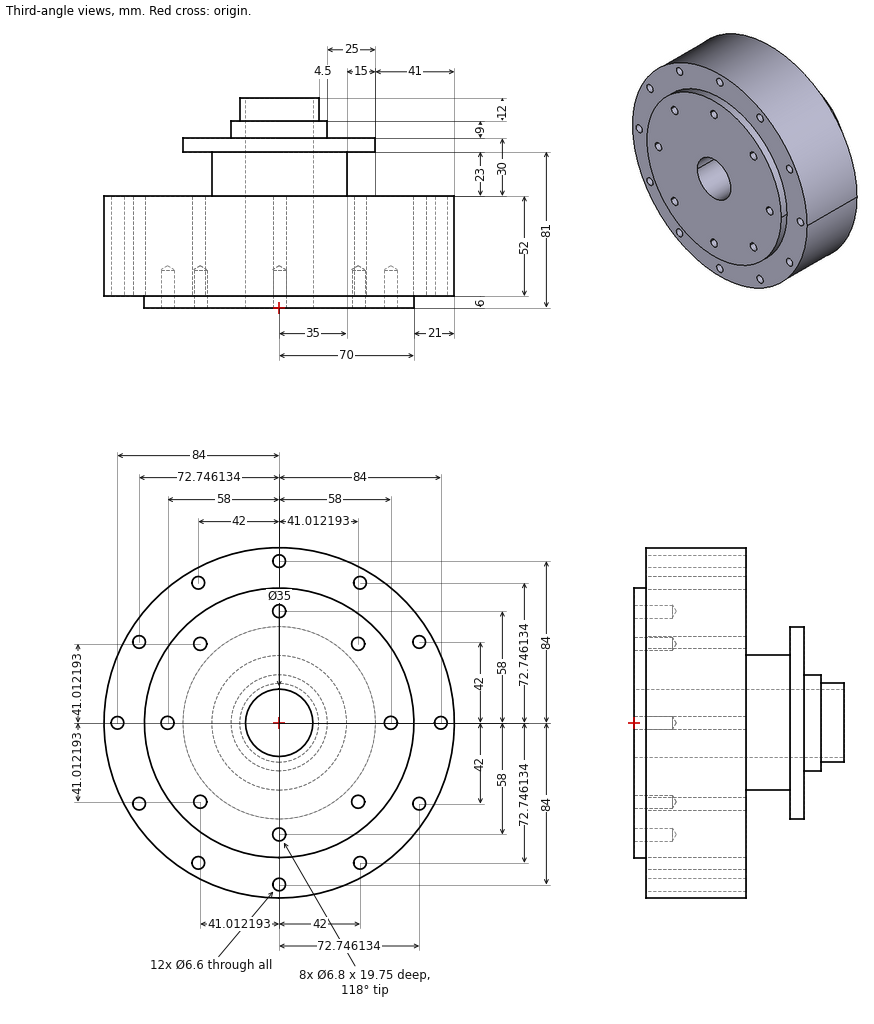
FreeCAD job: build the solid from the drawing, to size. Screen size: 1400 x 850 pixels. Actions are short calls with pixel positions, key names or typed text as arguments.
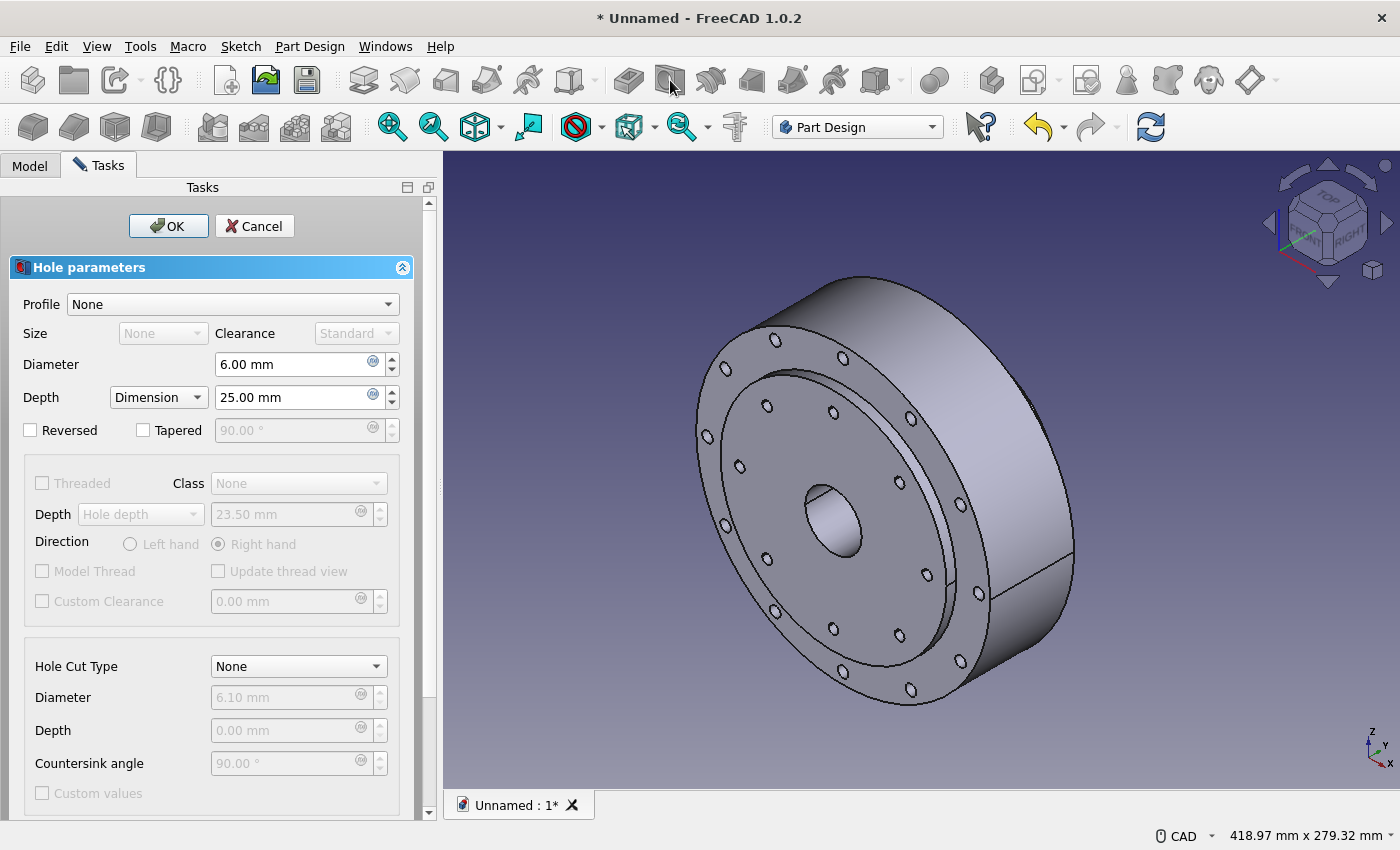
triple_click(300, 364)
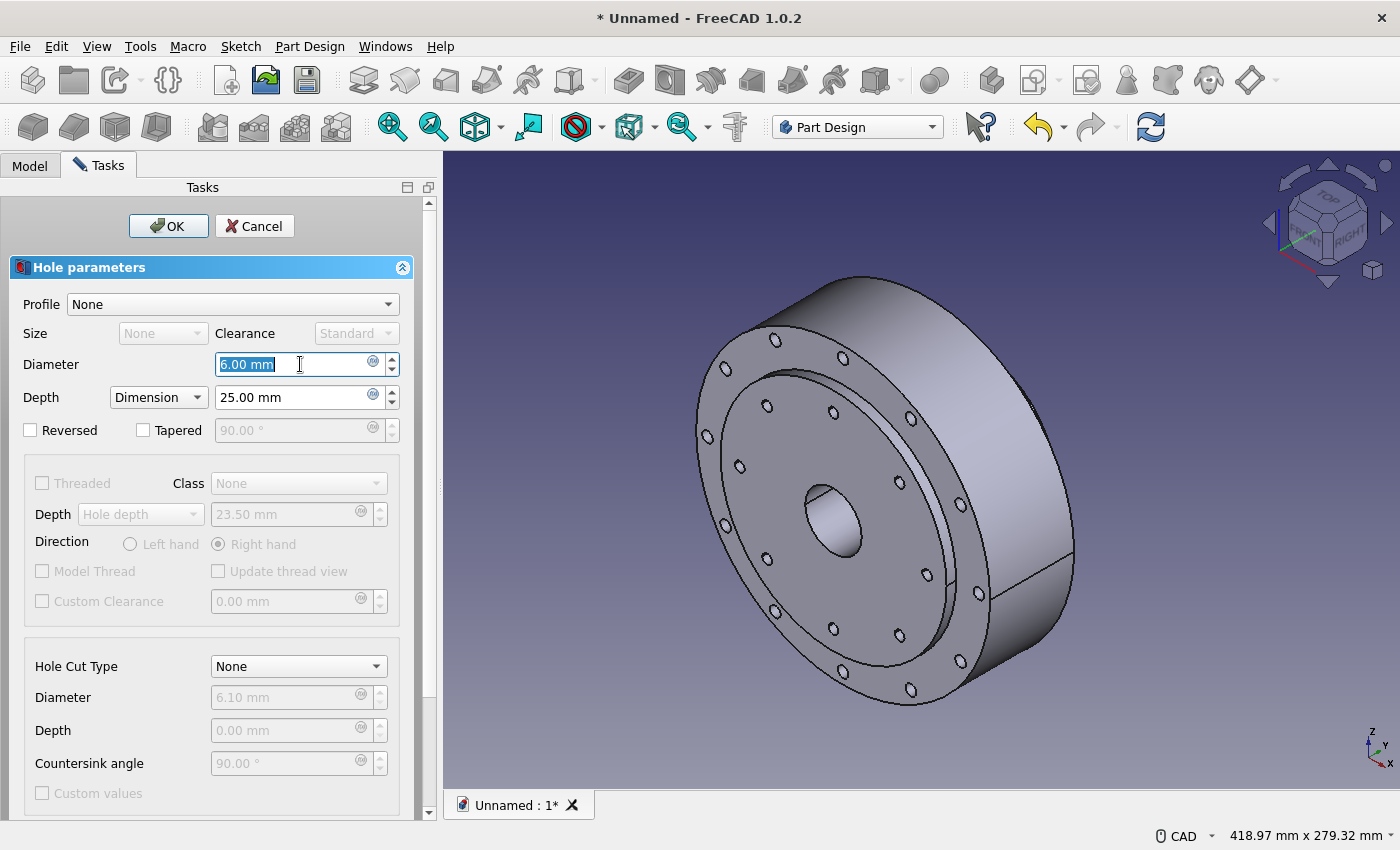
text(6.8)
key(Tab)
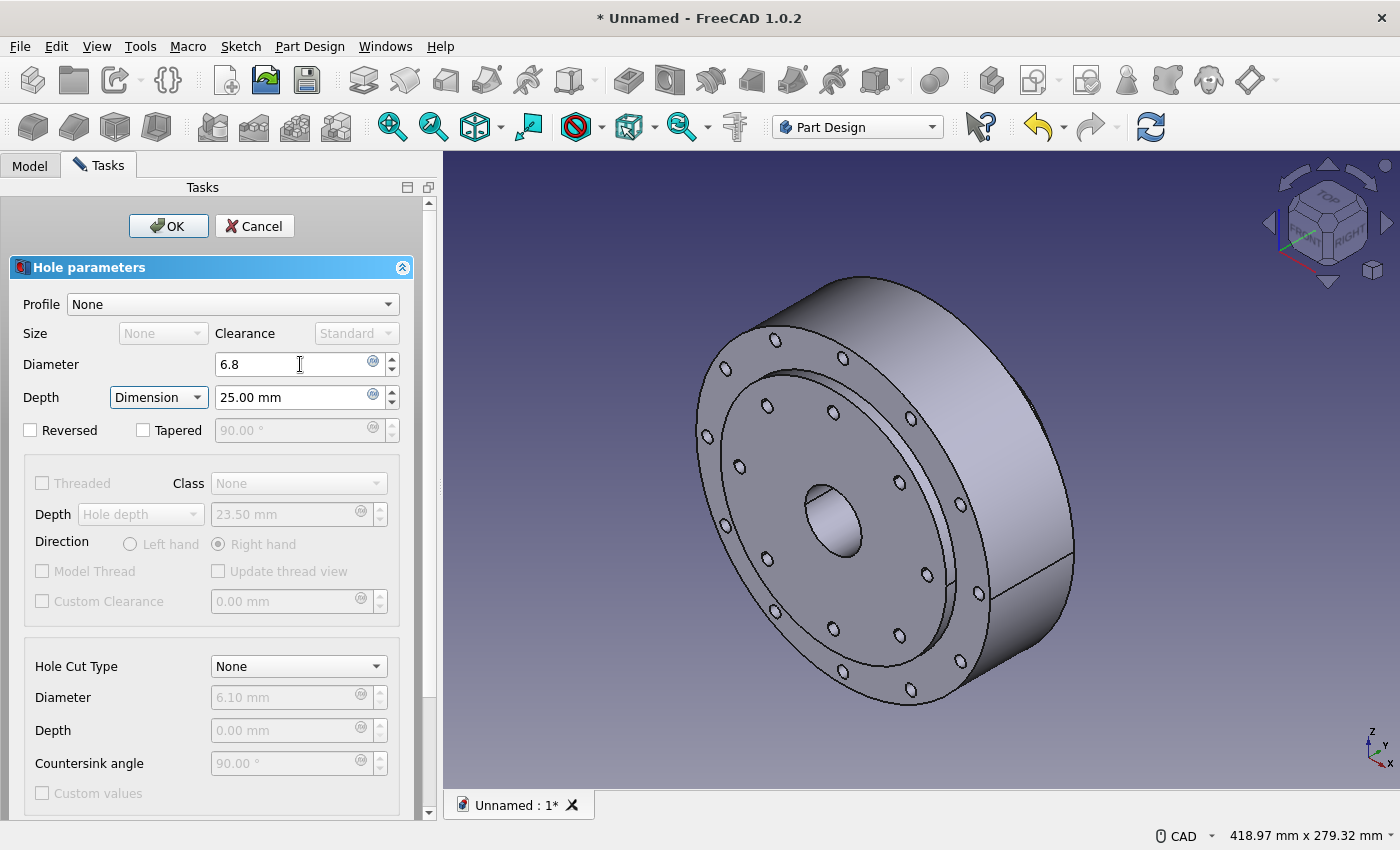
triple_click(300, 398)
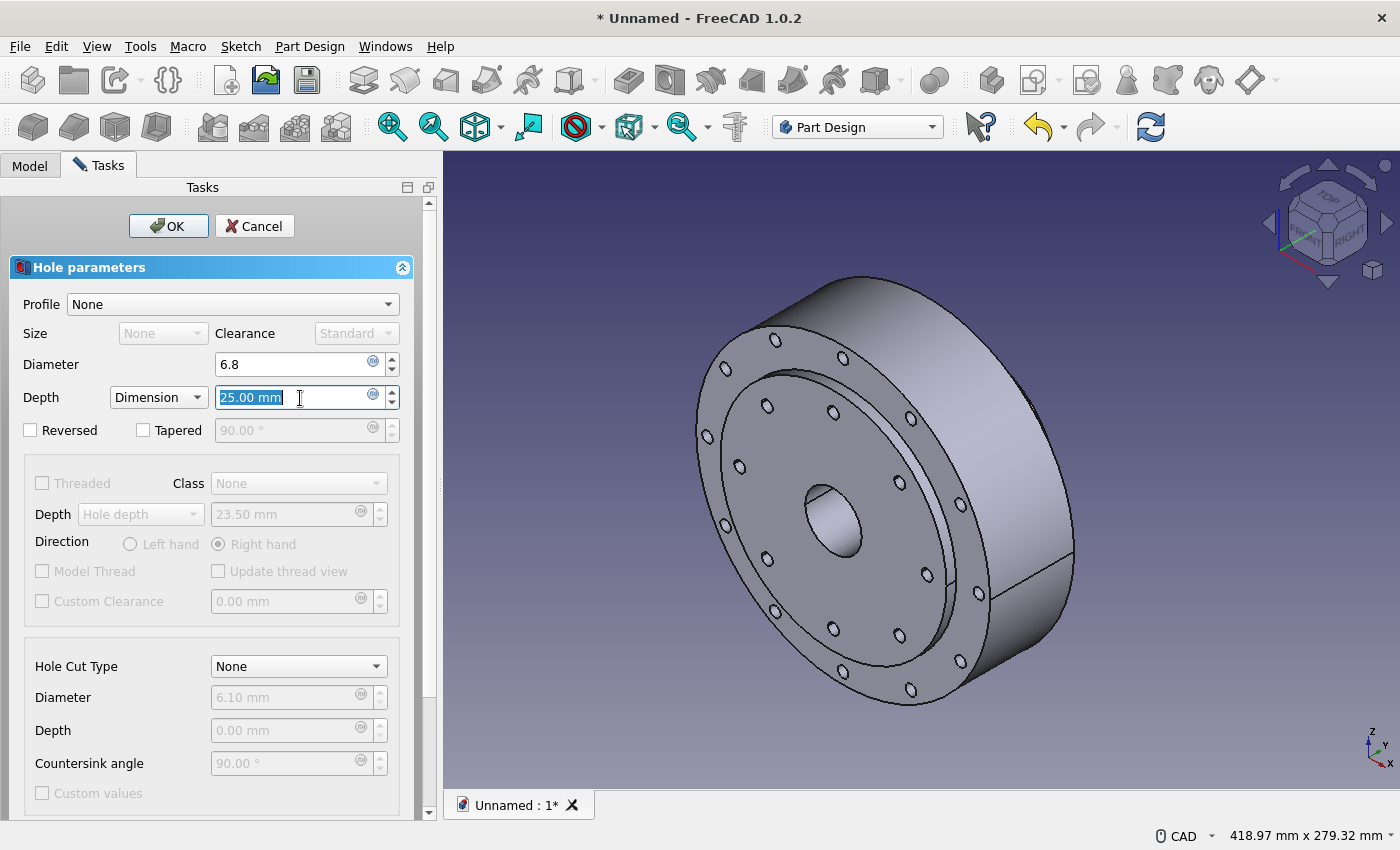
text(19.75)
key(Tab)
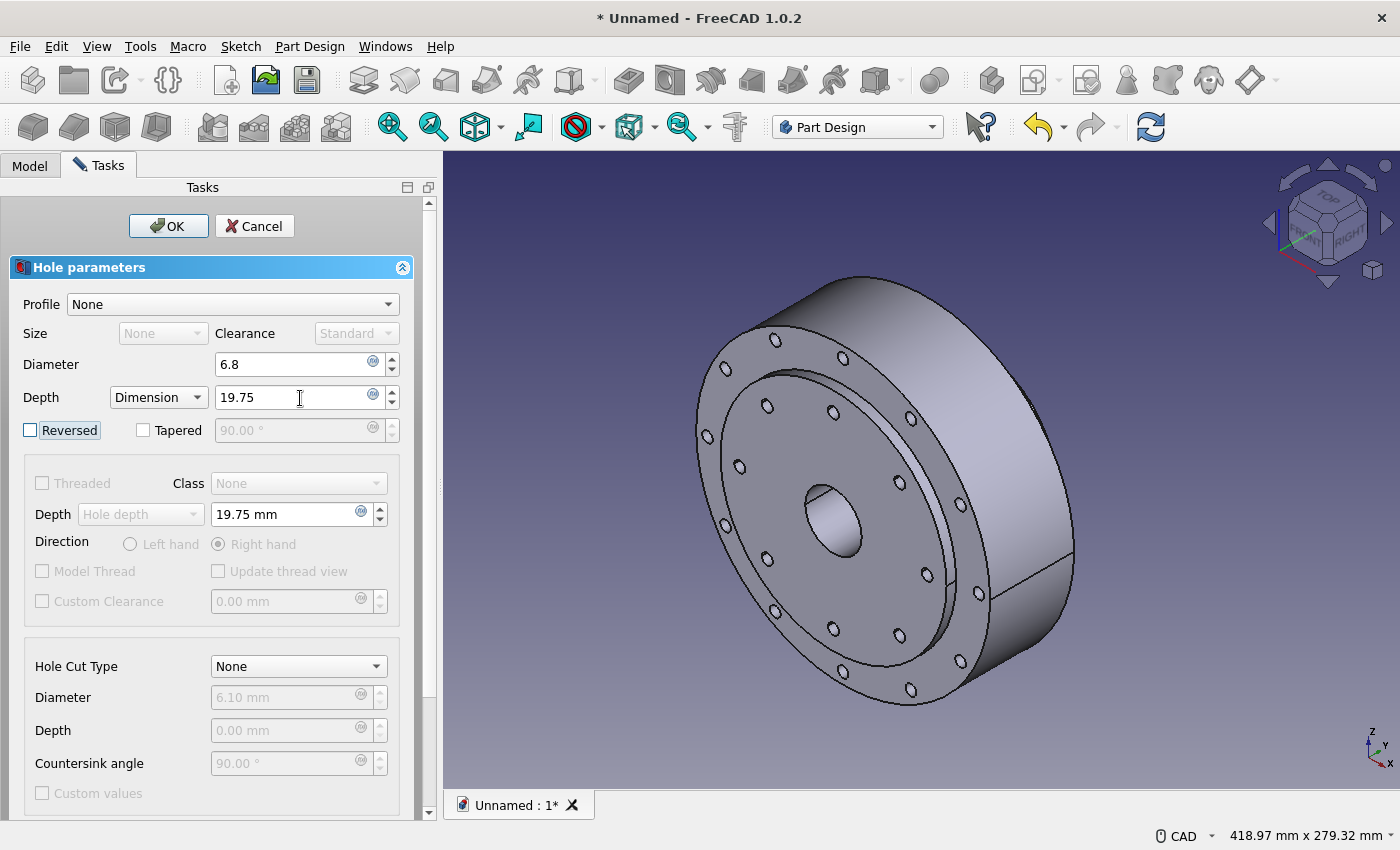
click(169, 226)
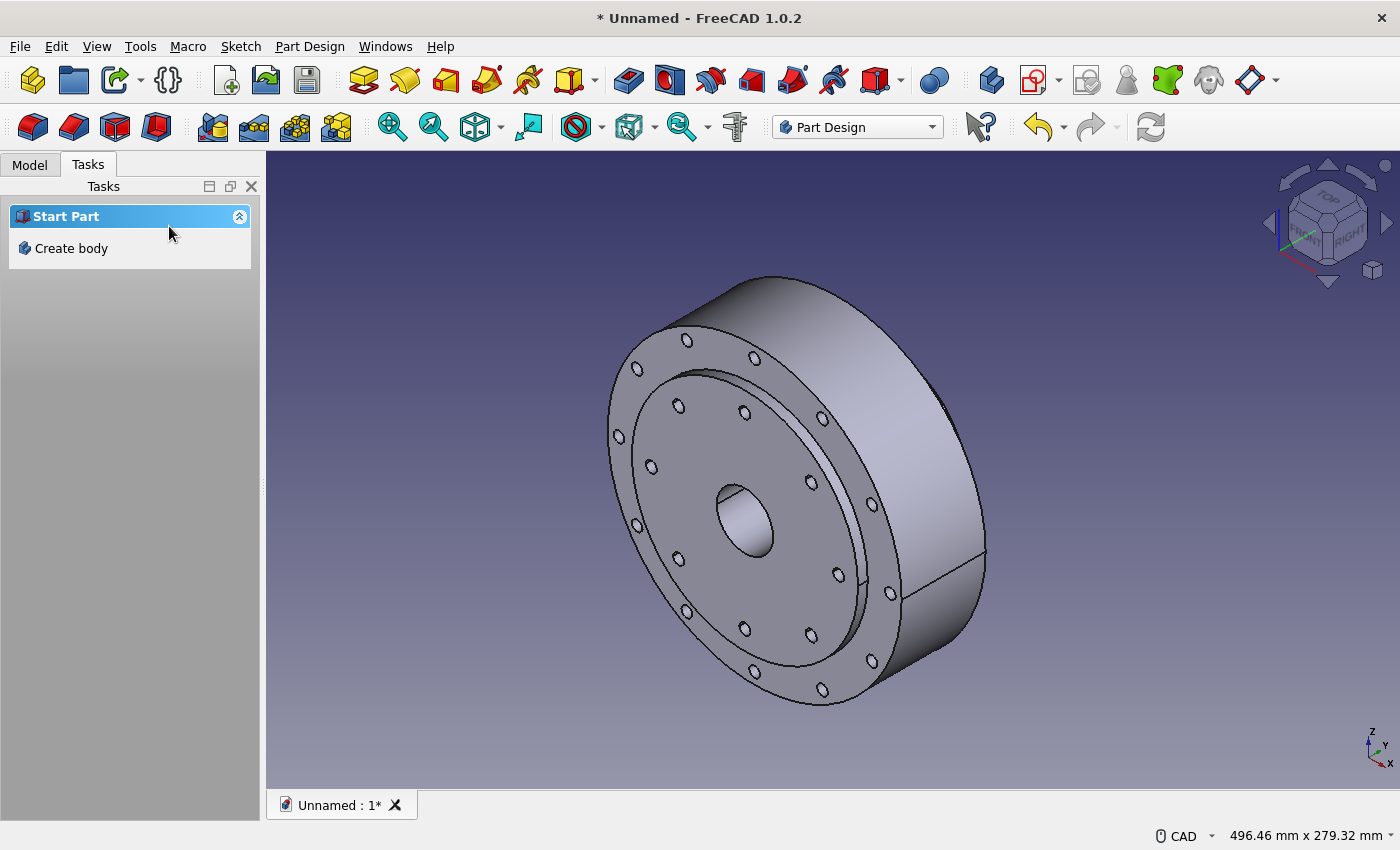
click(1032, 80)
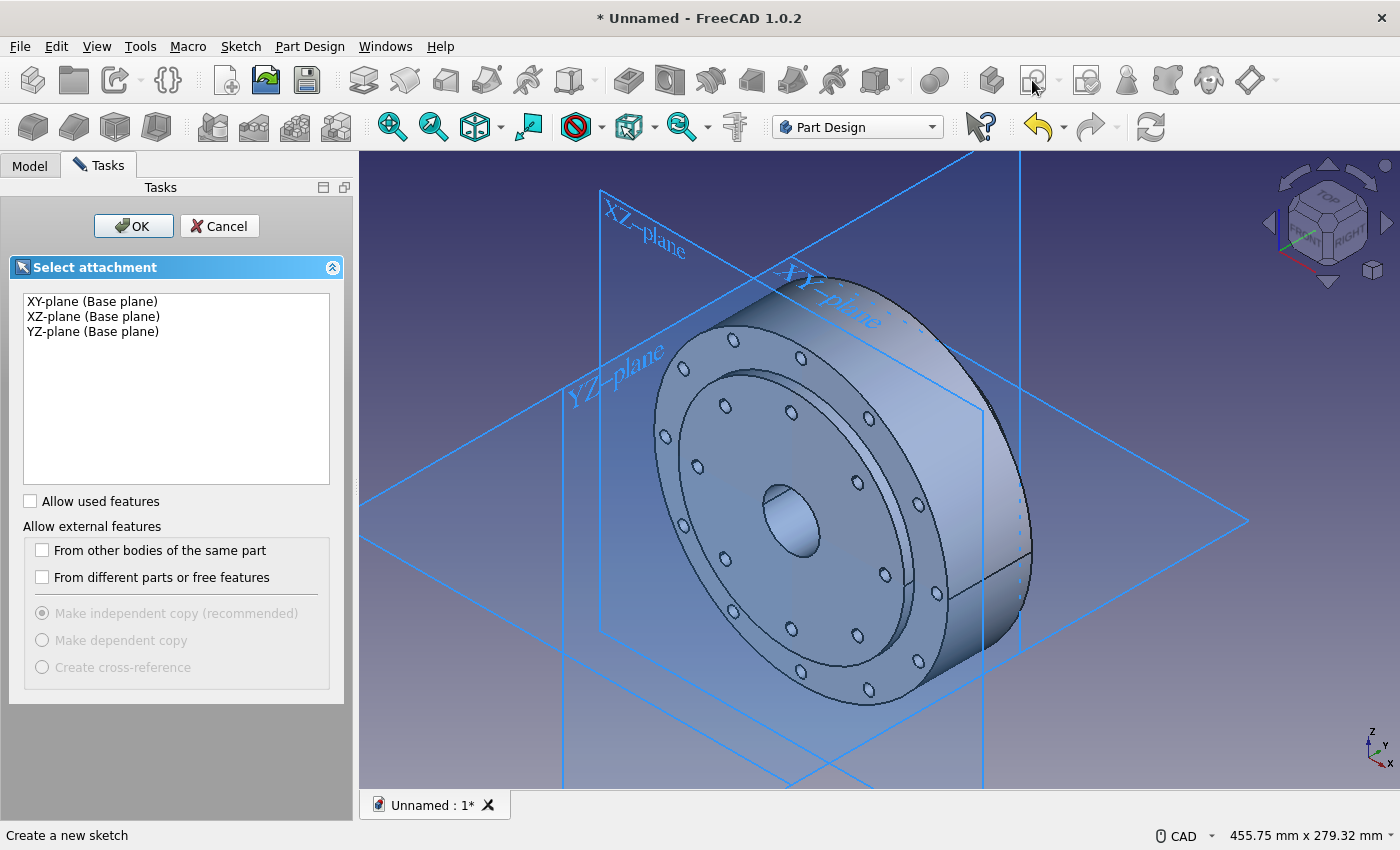
click(84, 302)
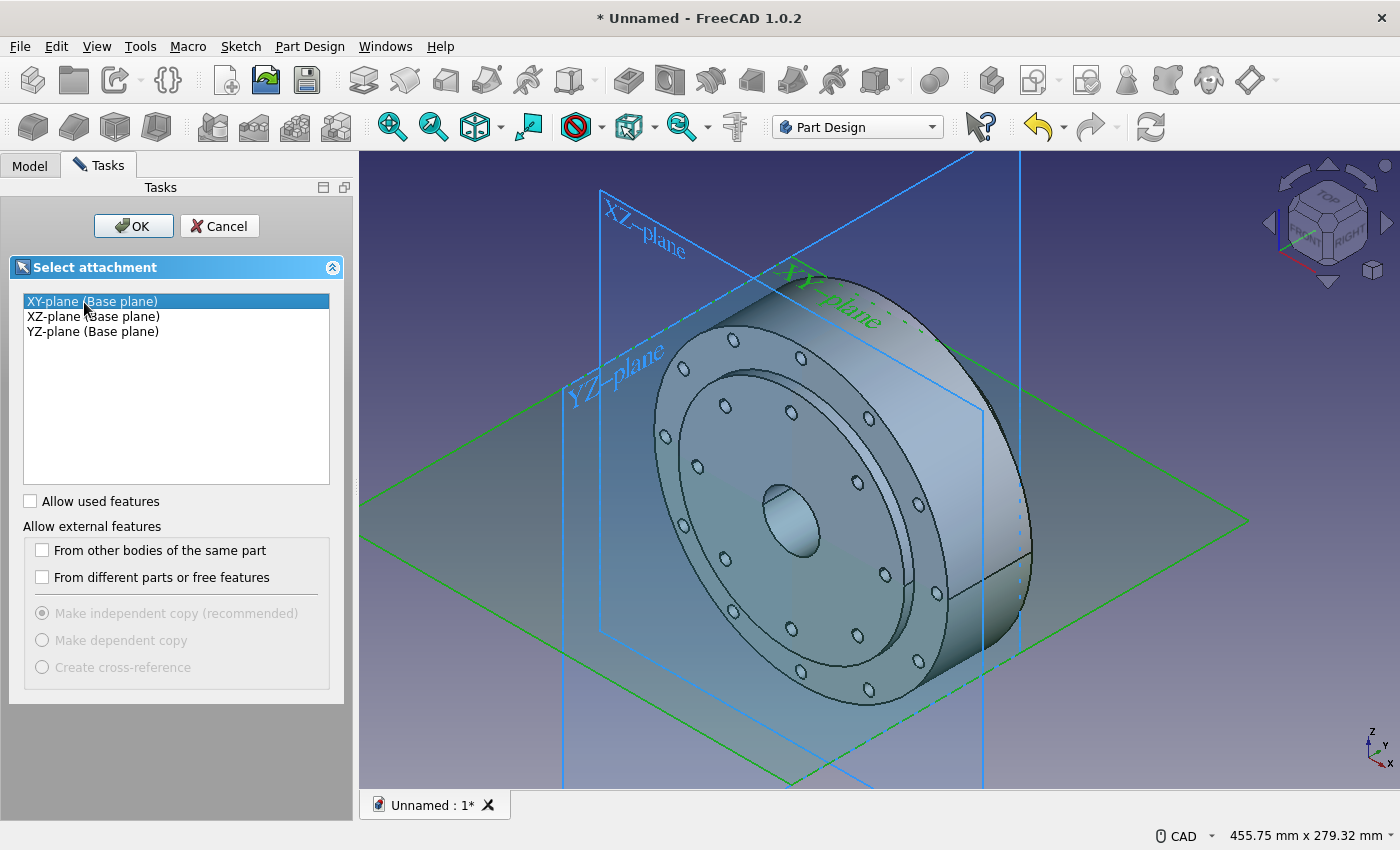
click(134, 226)